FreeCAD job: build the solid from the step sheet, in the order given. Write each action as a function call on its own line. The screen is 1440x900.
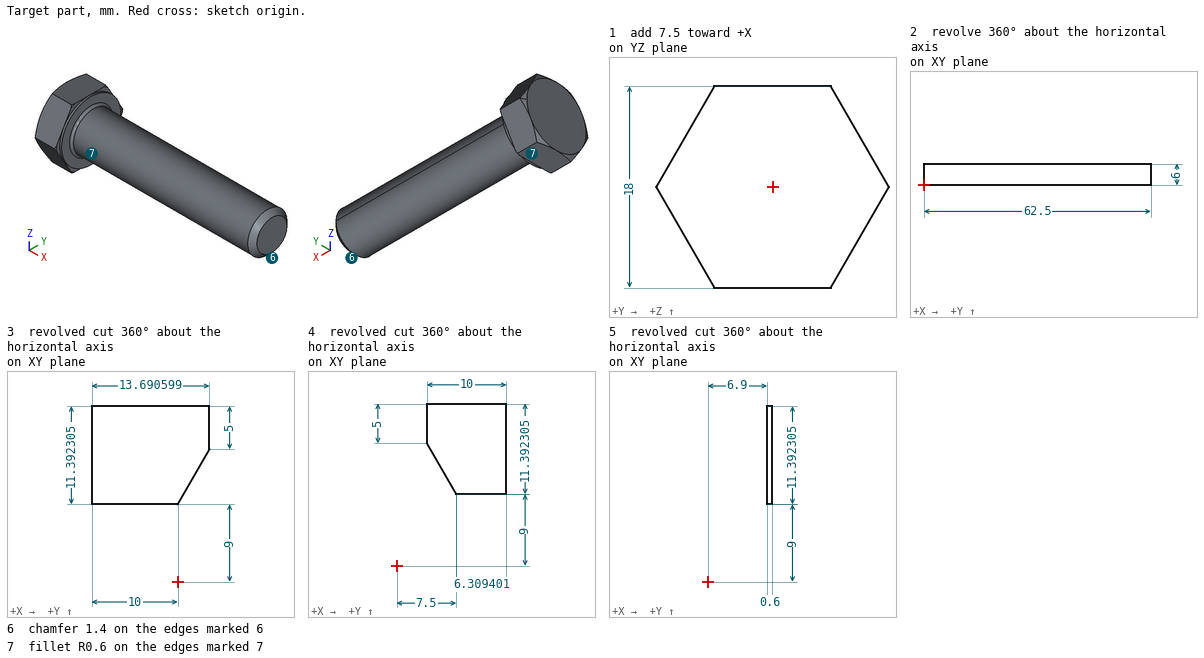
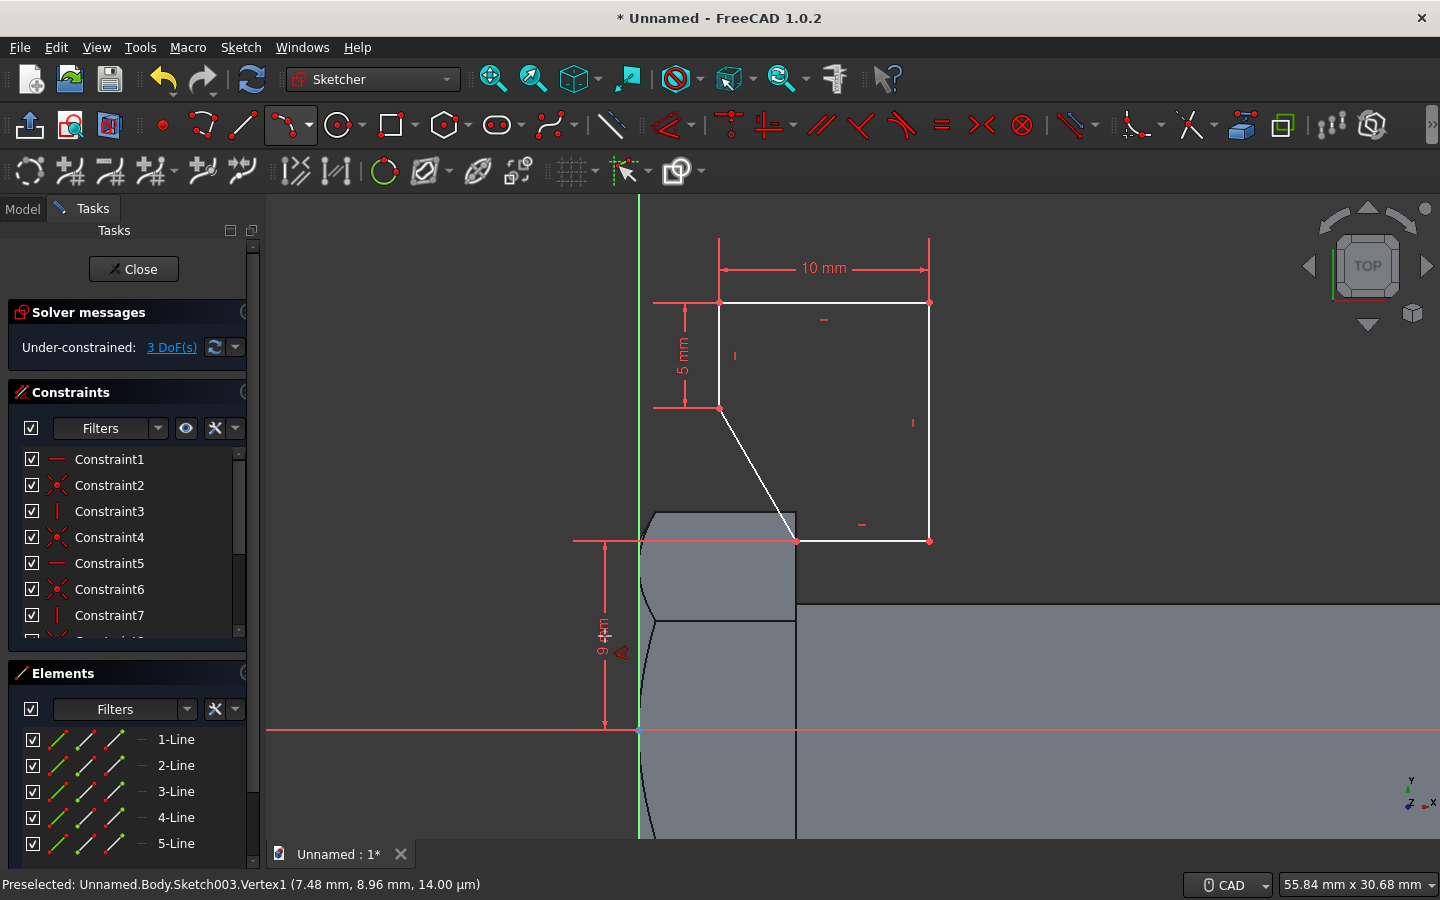
click(796, 541)
click(717, 764)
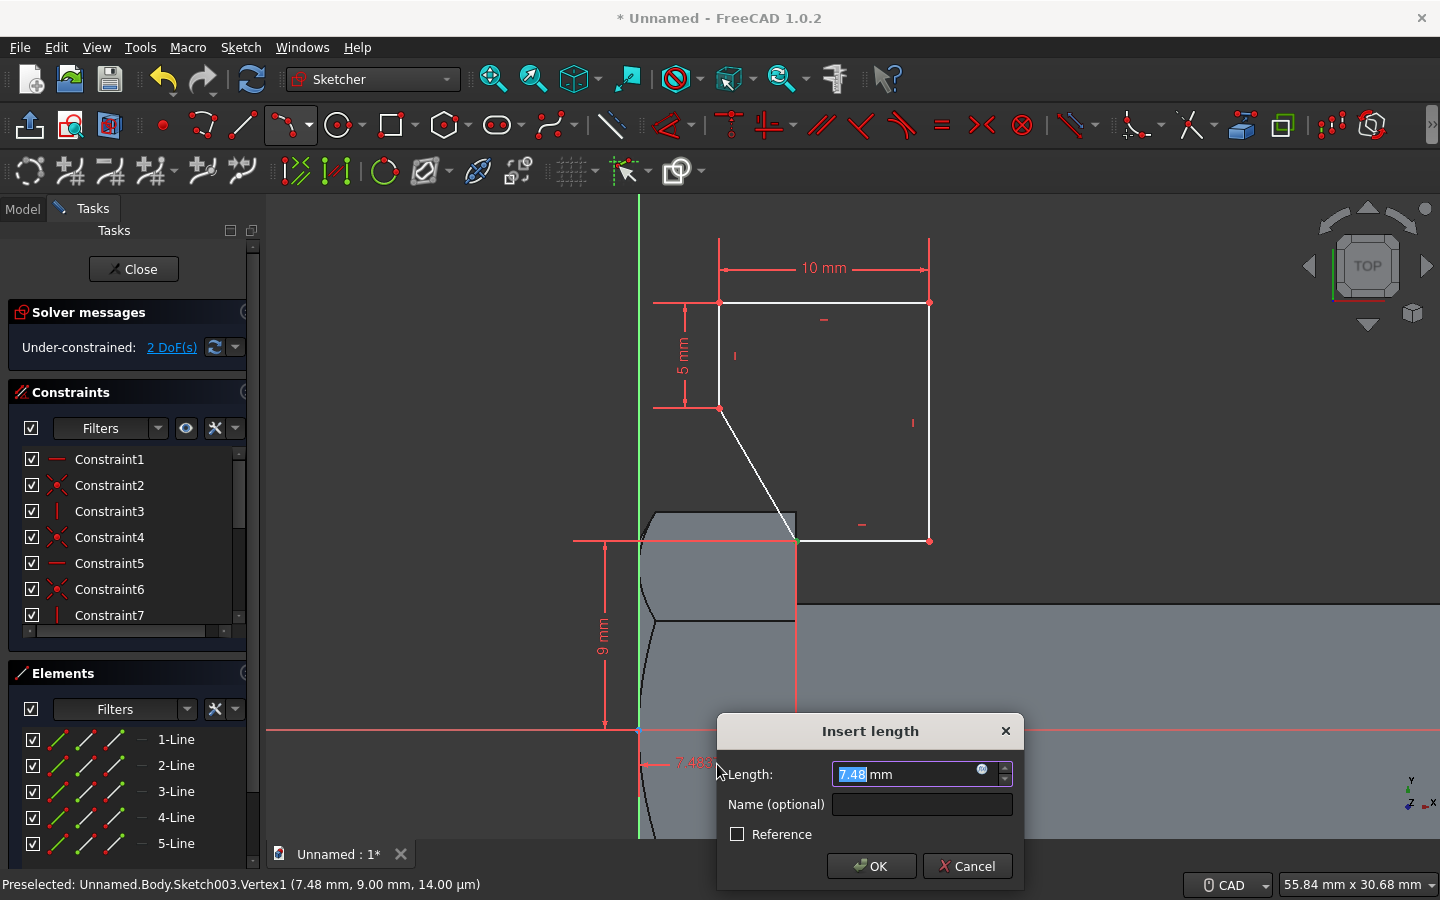
text(7.5)
key(Return)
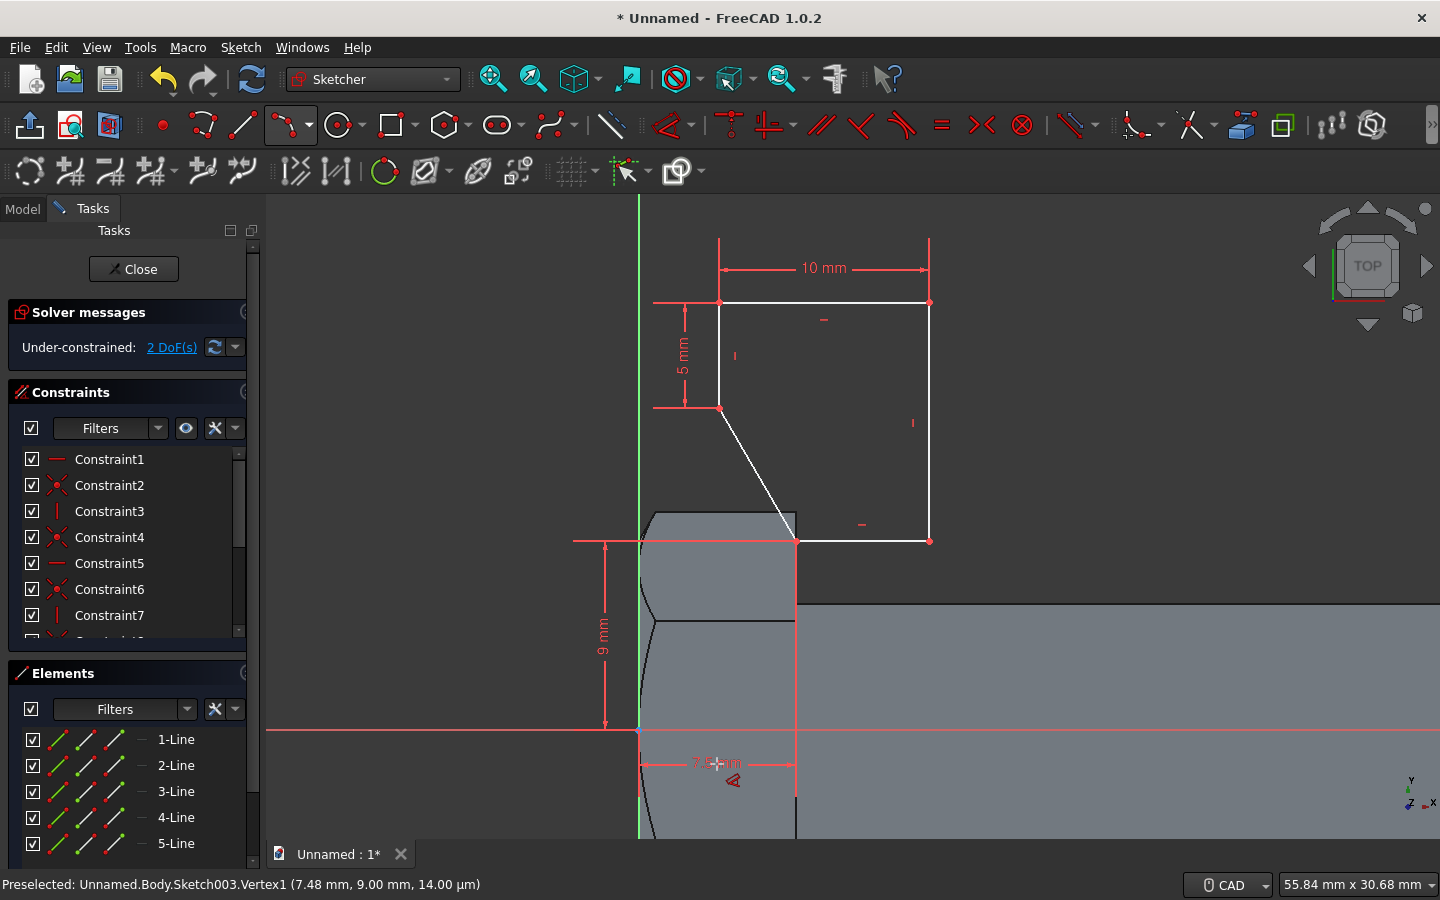
click(836, 541)
click(863, 575)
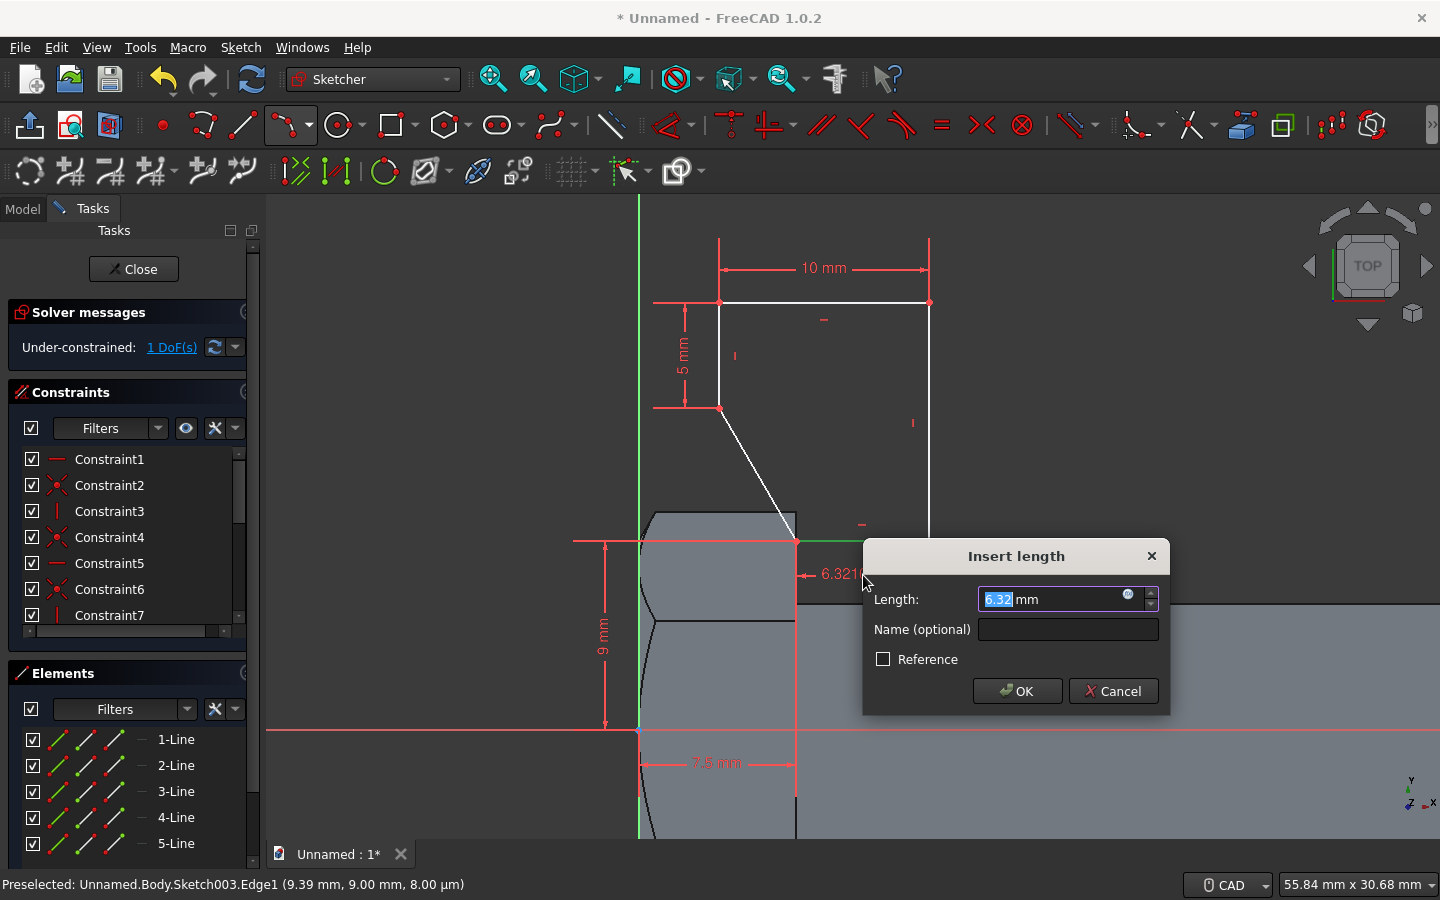
text(6.309401)
key(Return)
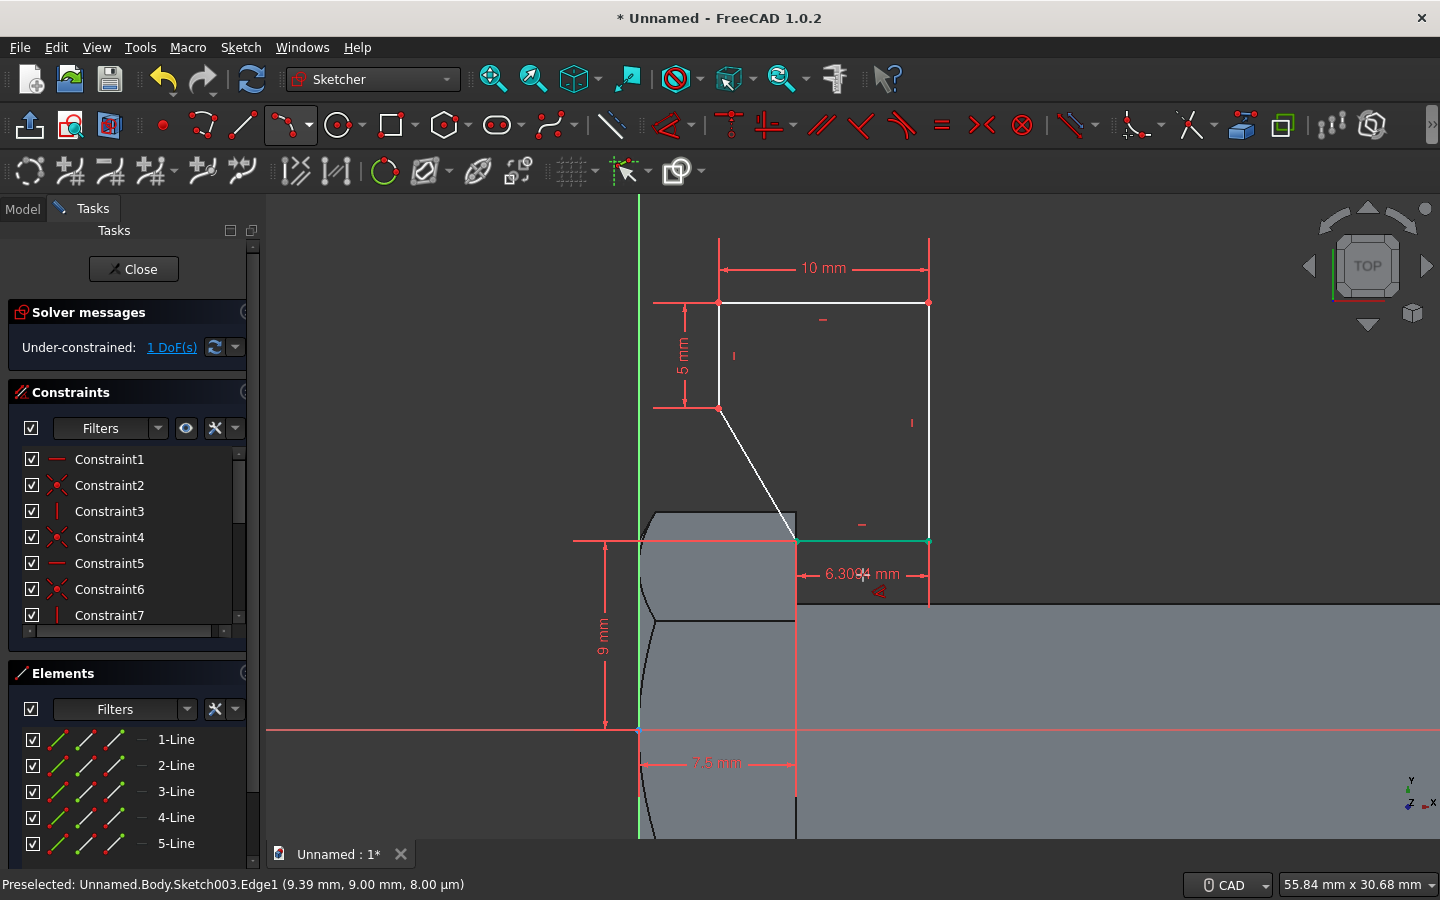
click(929, 470)
click(963, 422)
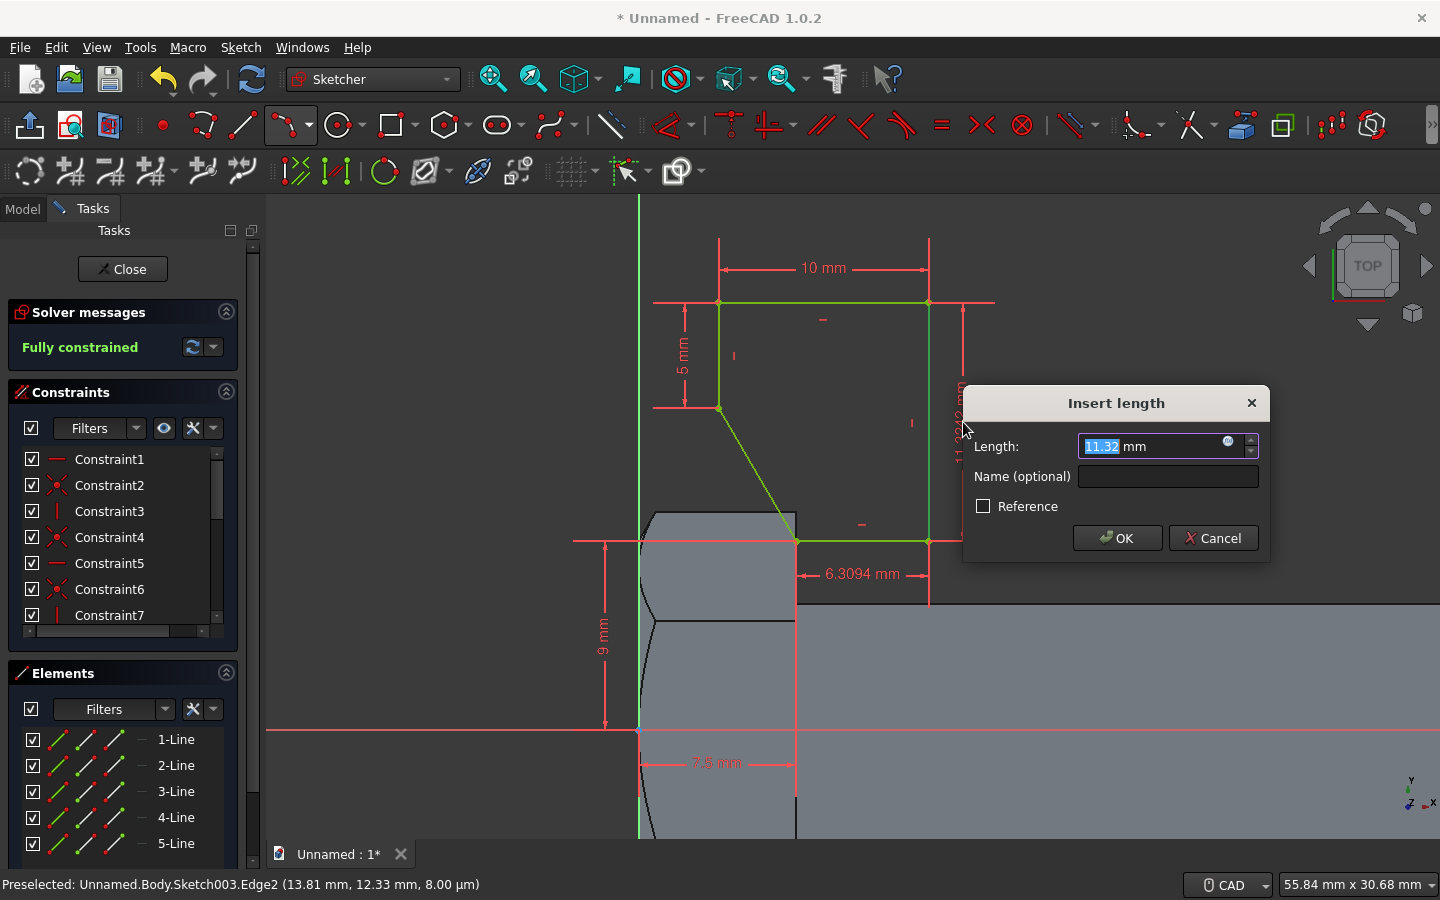
text(11.392305)
key(Return)
key(Escape)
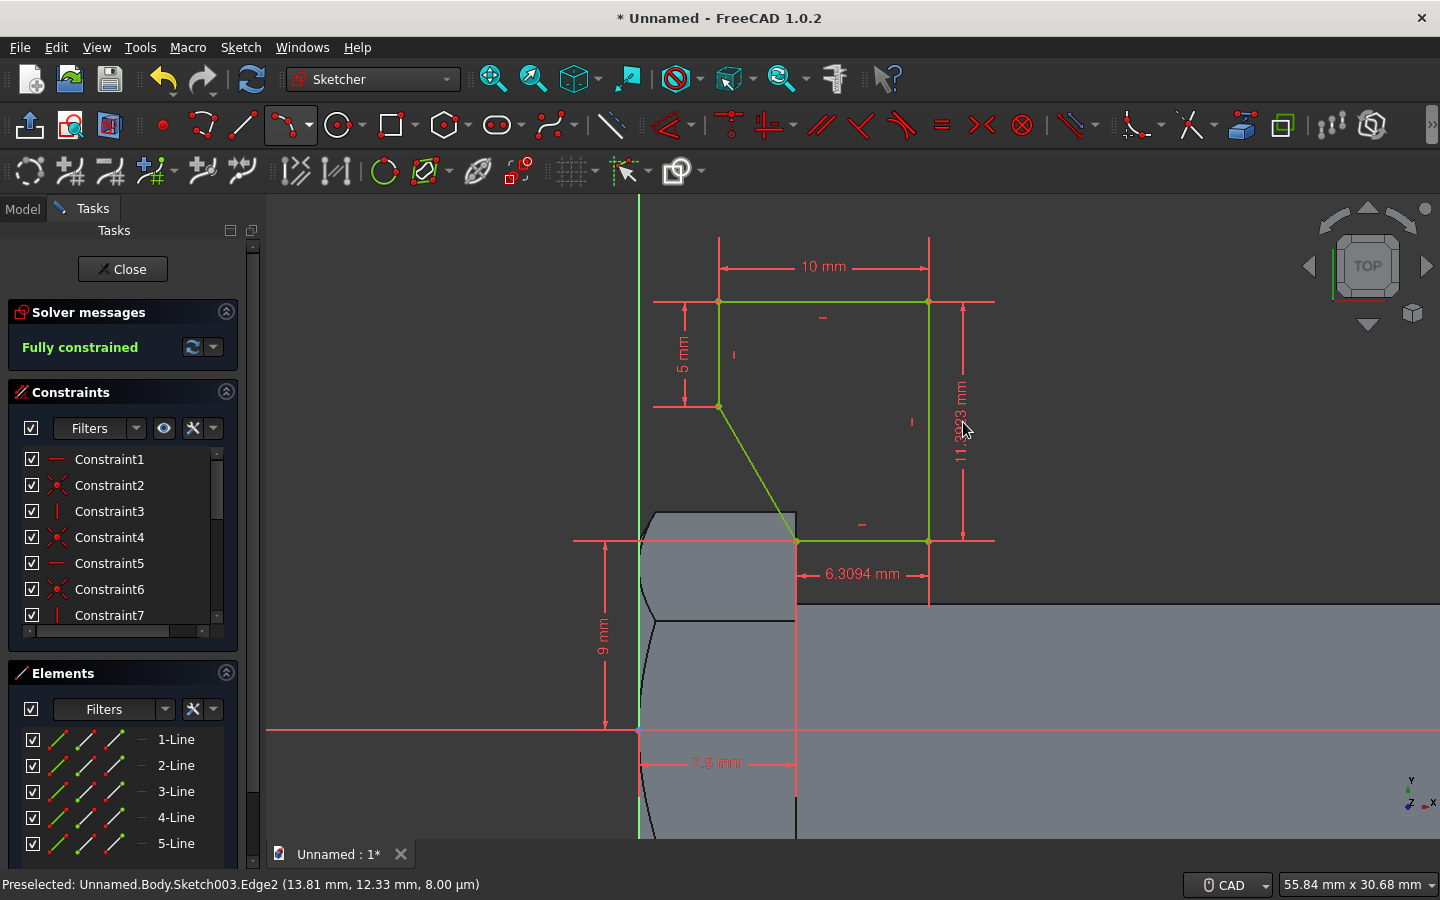
click(123, 269)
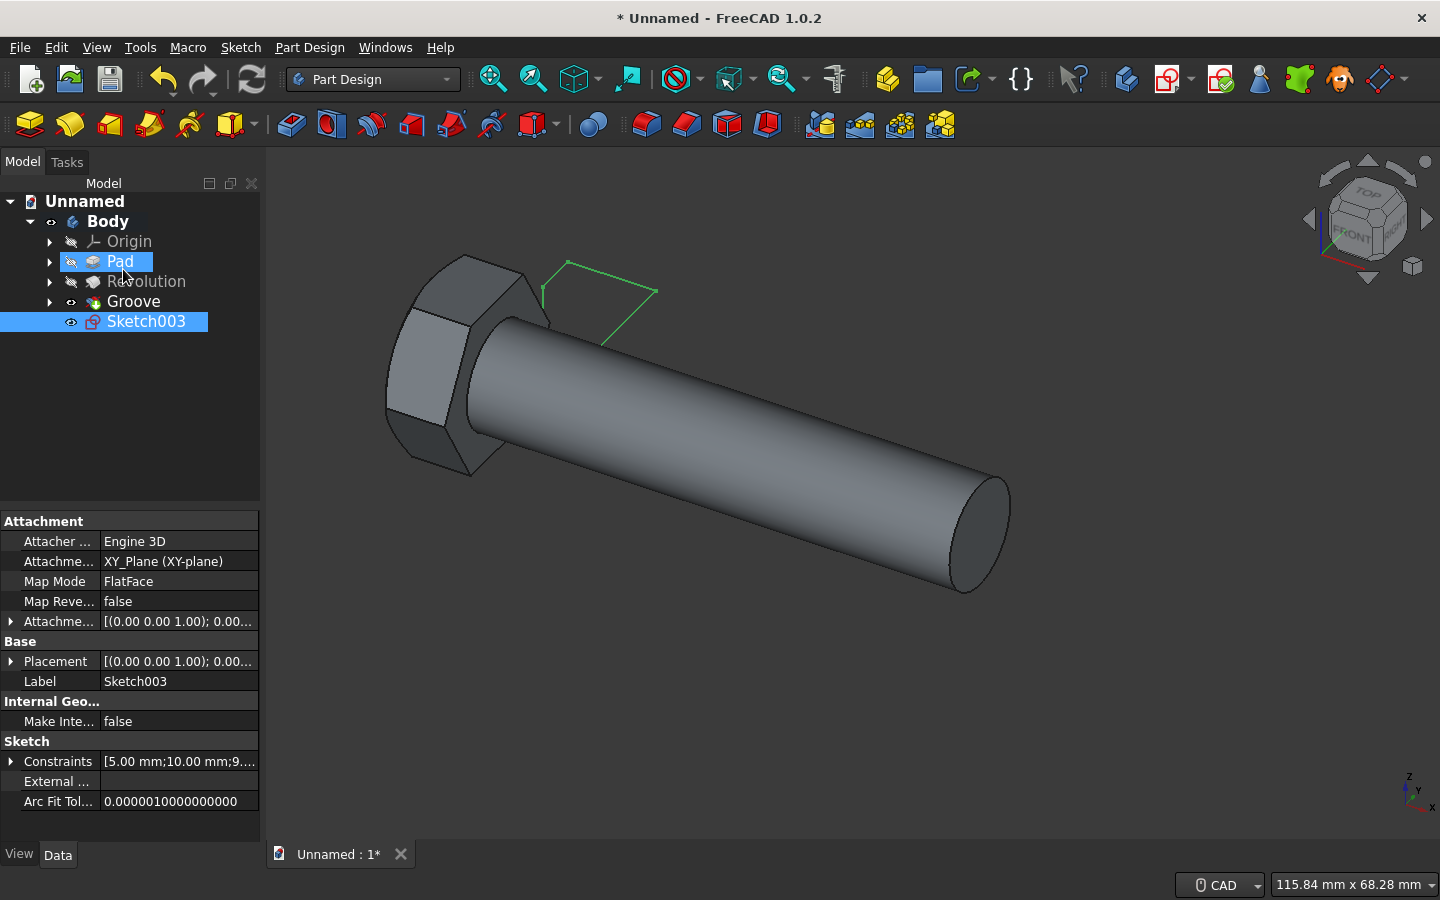
click(372, 124)